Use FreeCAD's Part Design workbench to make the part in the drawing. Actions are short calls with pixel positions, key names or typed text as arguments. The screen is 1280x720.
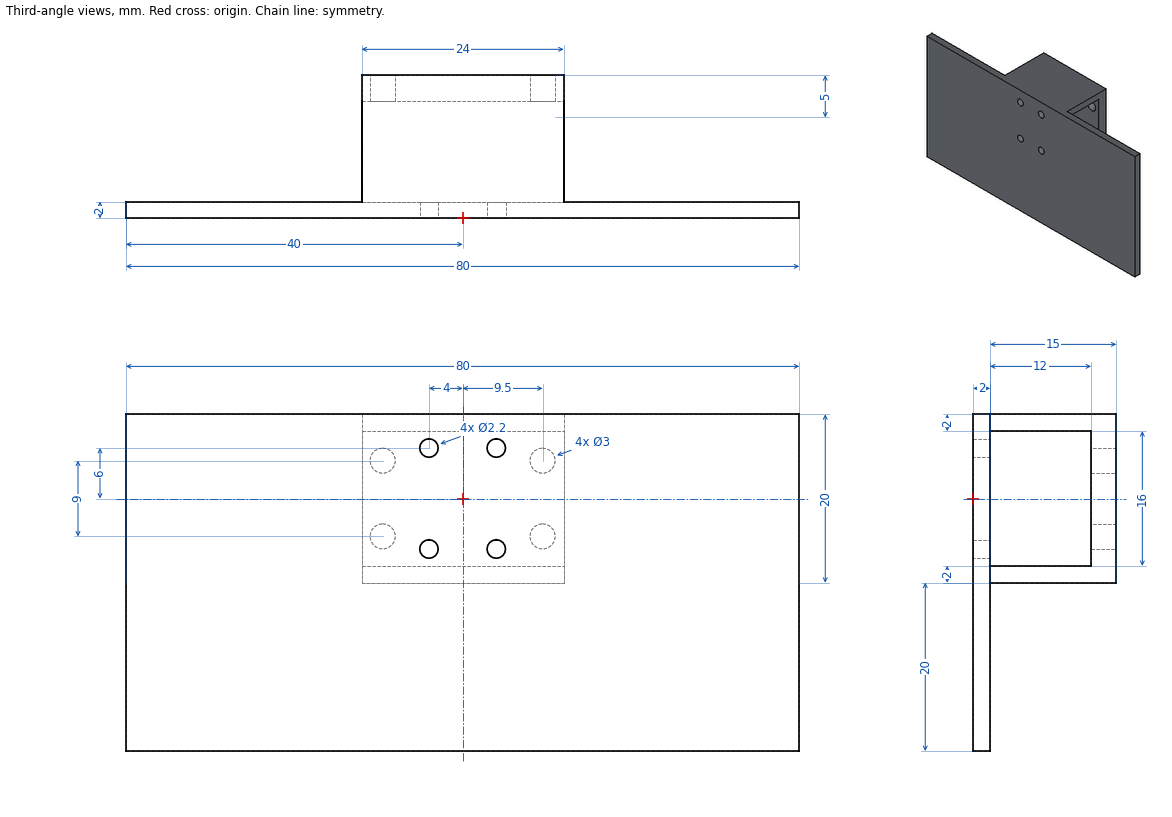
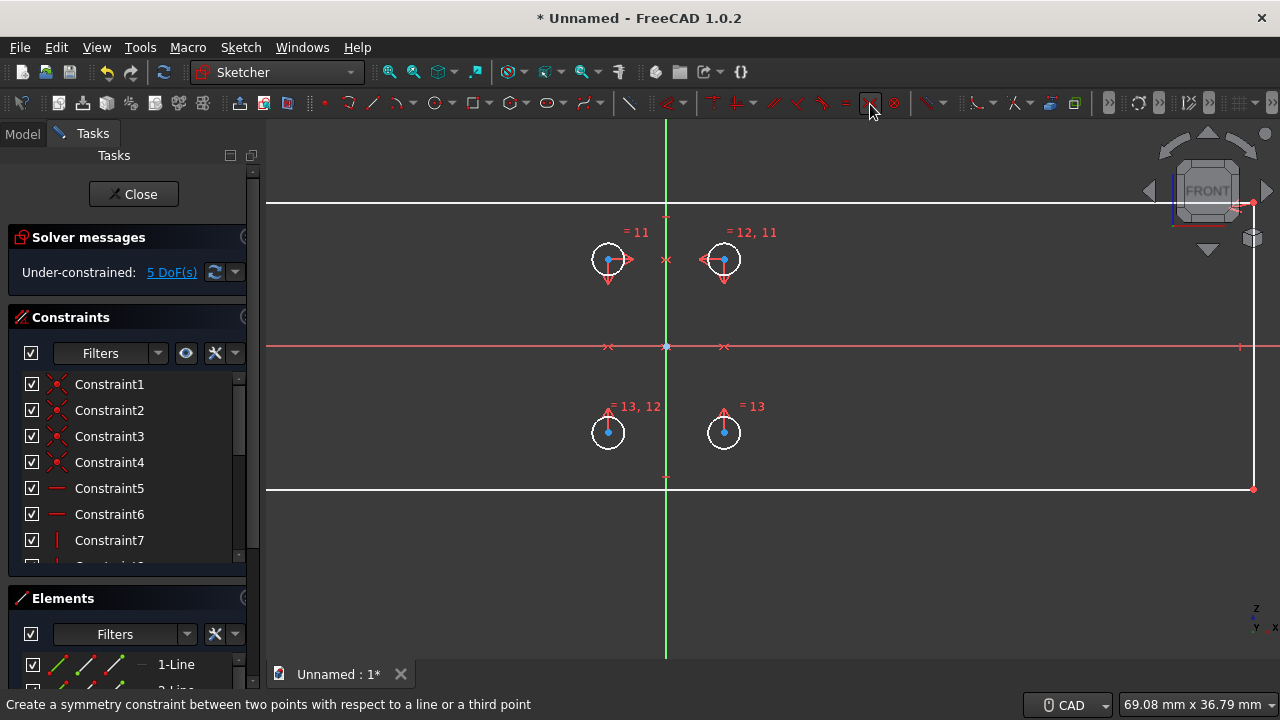
scroll(620, 248, up, 2)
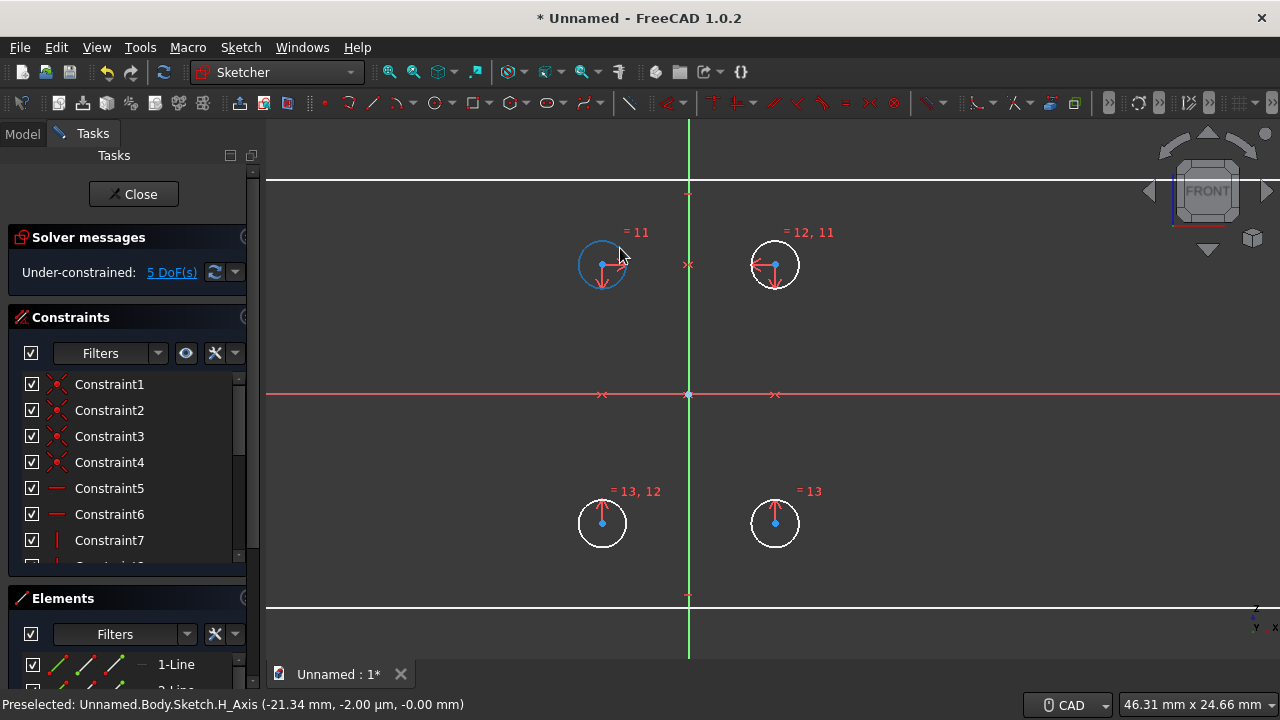
click(619, 248)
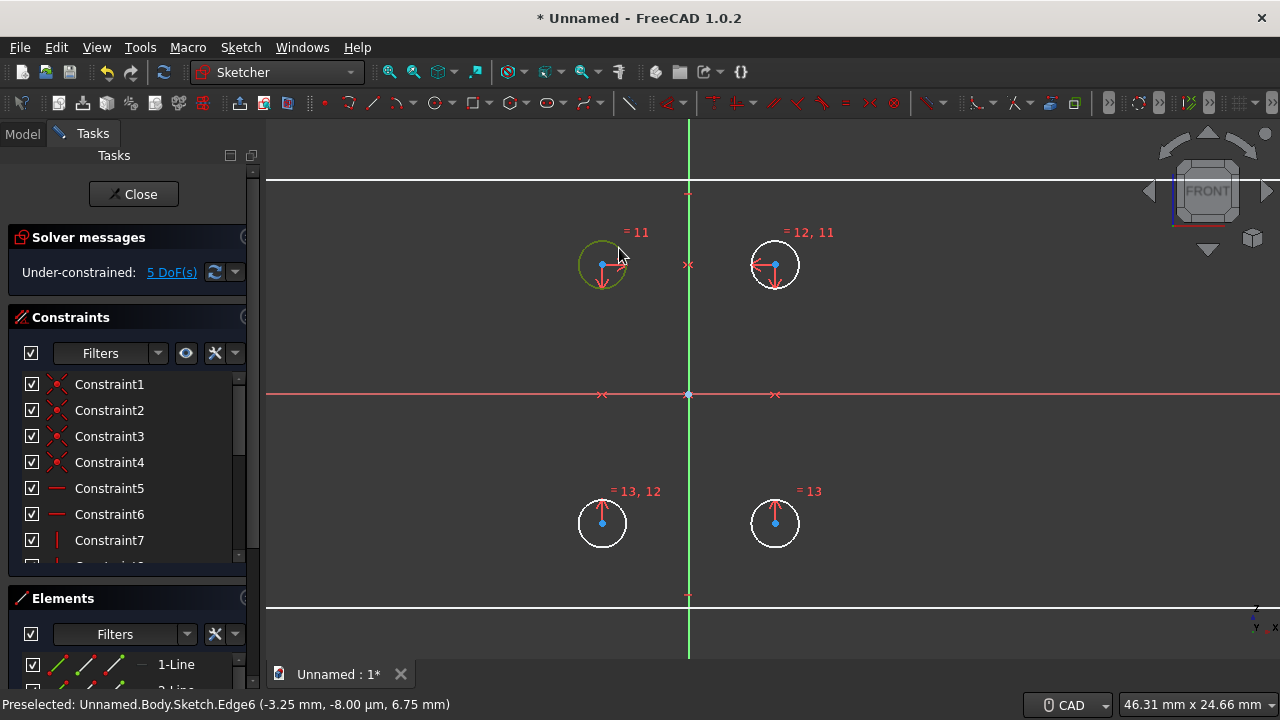
key(k)
key(o)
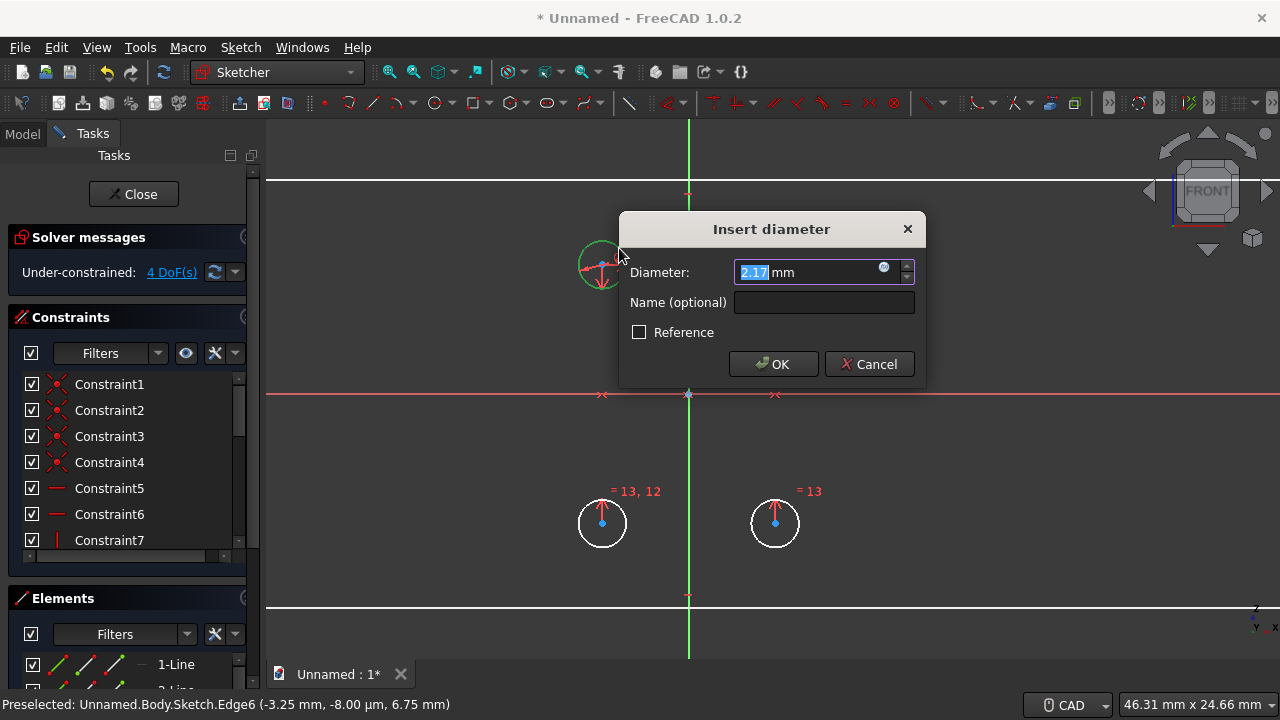
text(2.2)
key(Return)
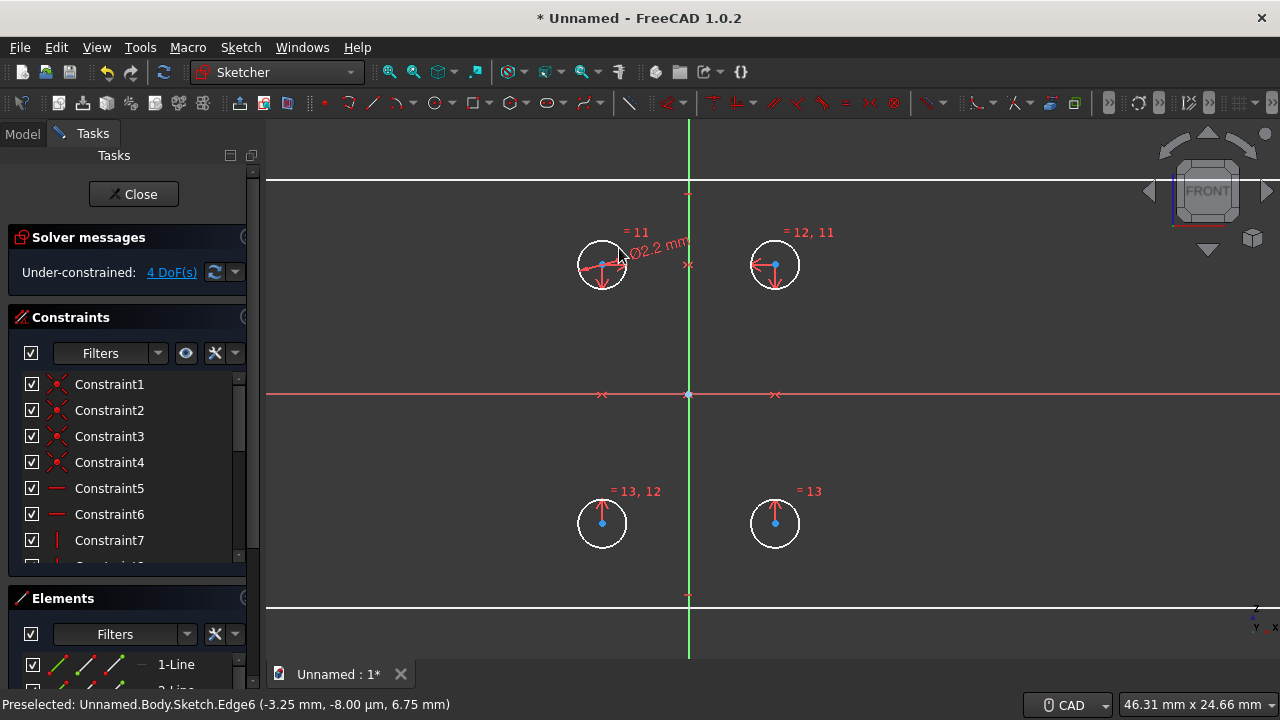
click(602, 265)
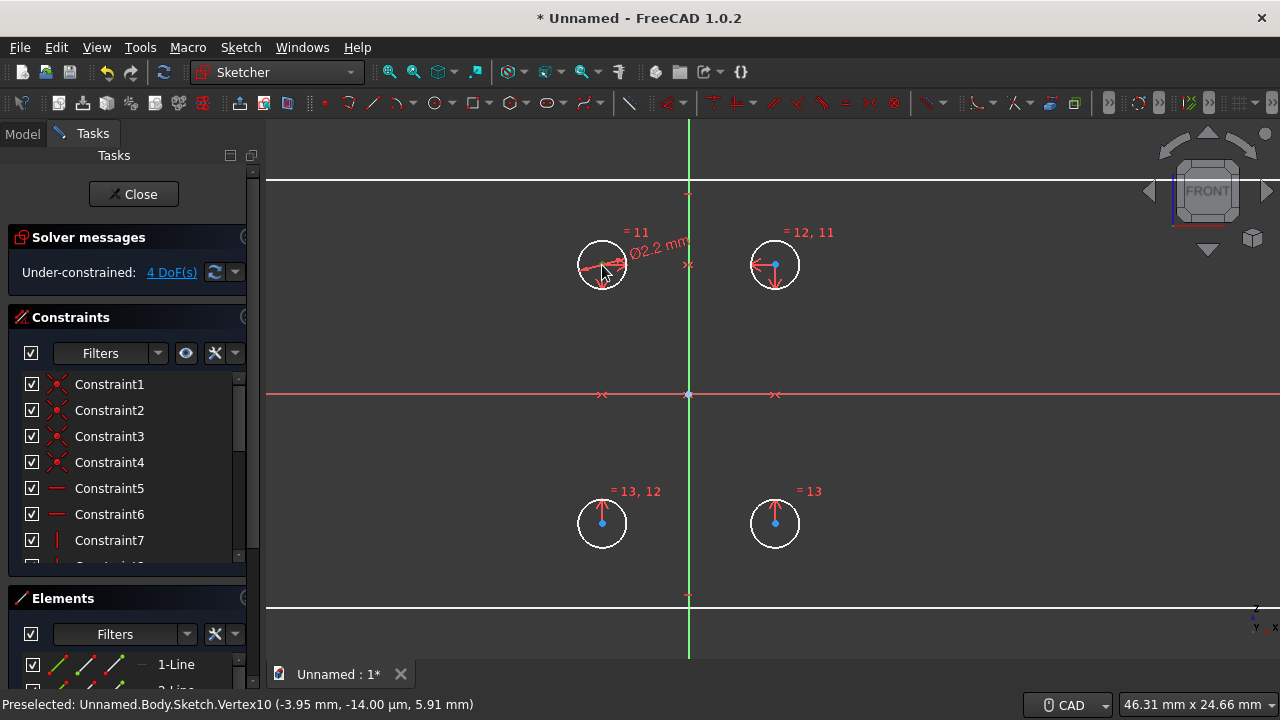
click(686, 104)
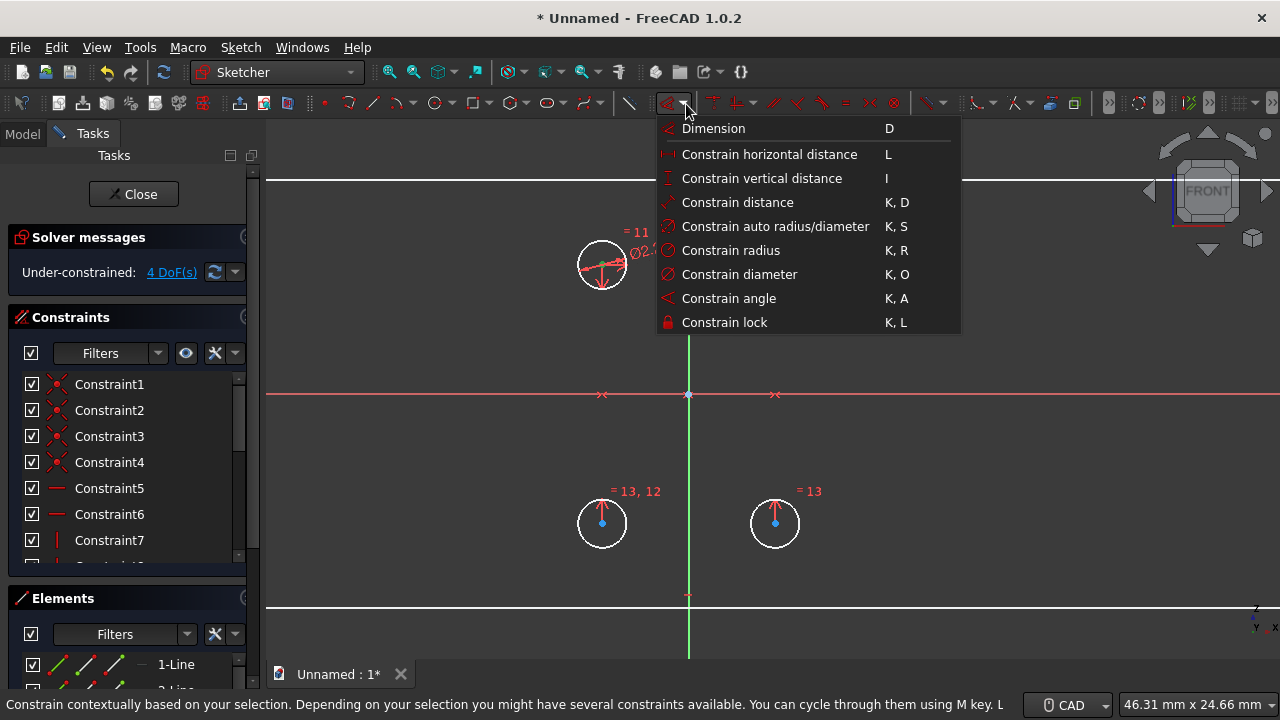
click(809, 154)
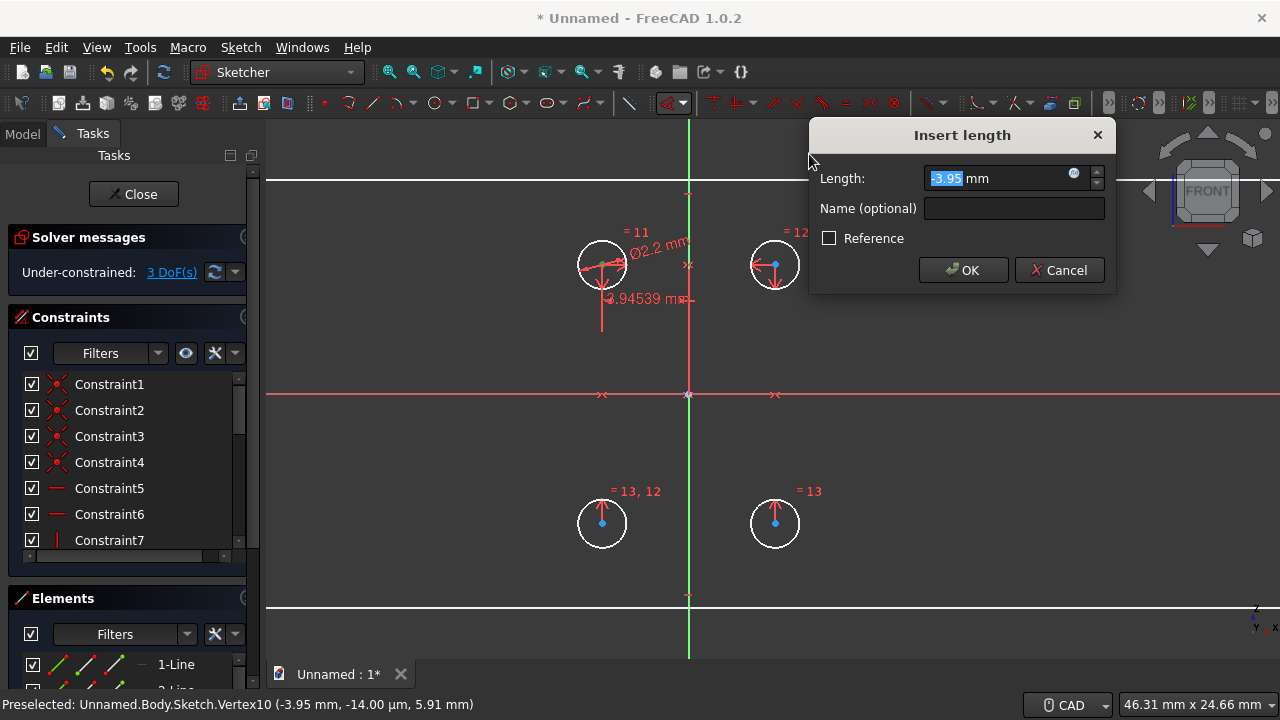
text(-4)
key(Return)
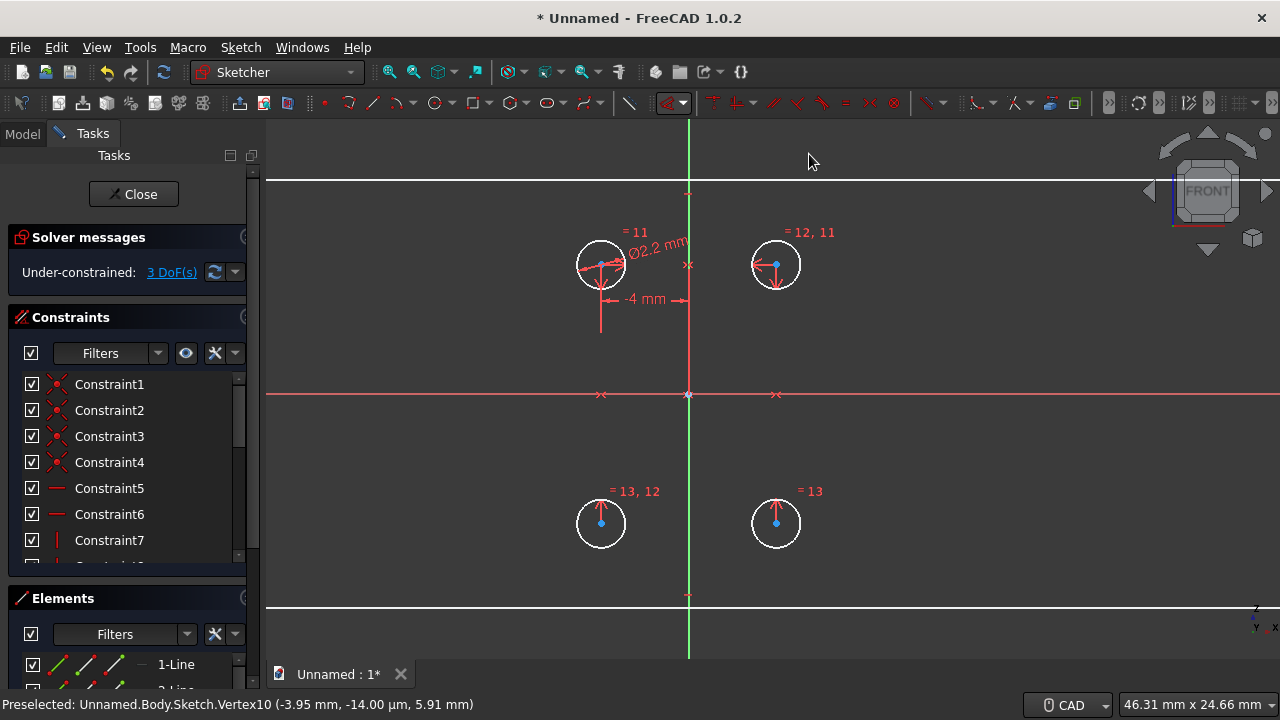
scroll(711, 387, down, 6)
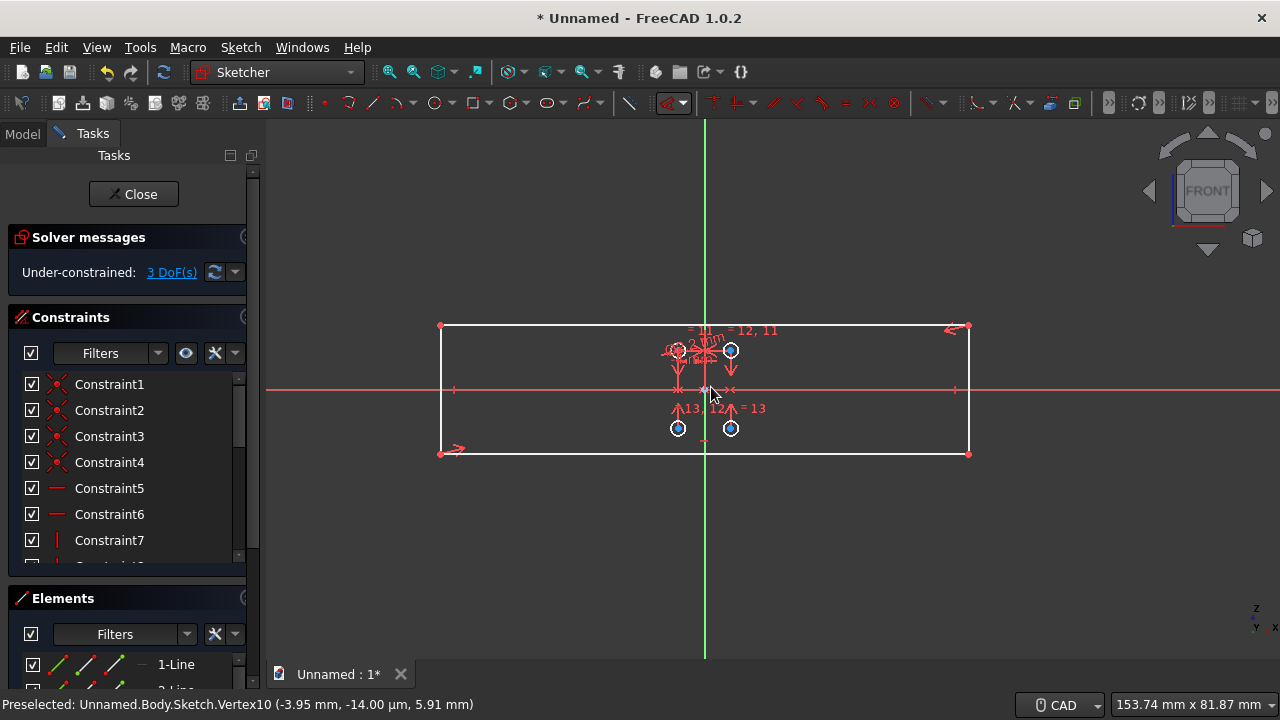
click(678, 351)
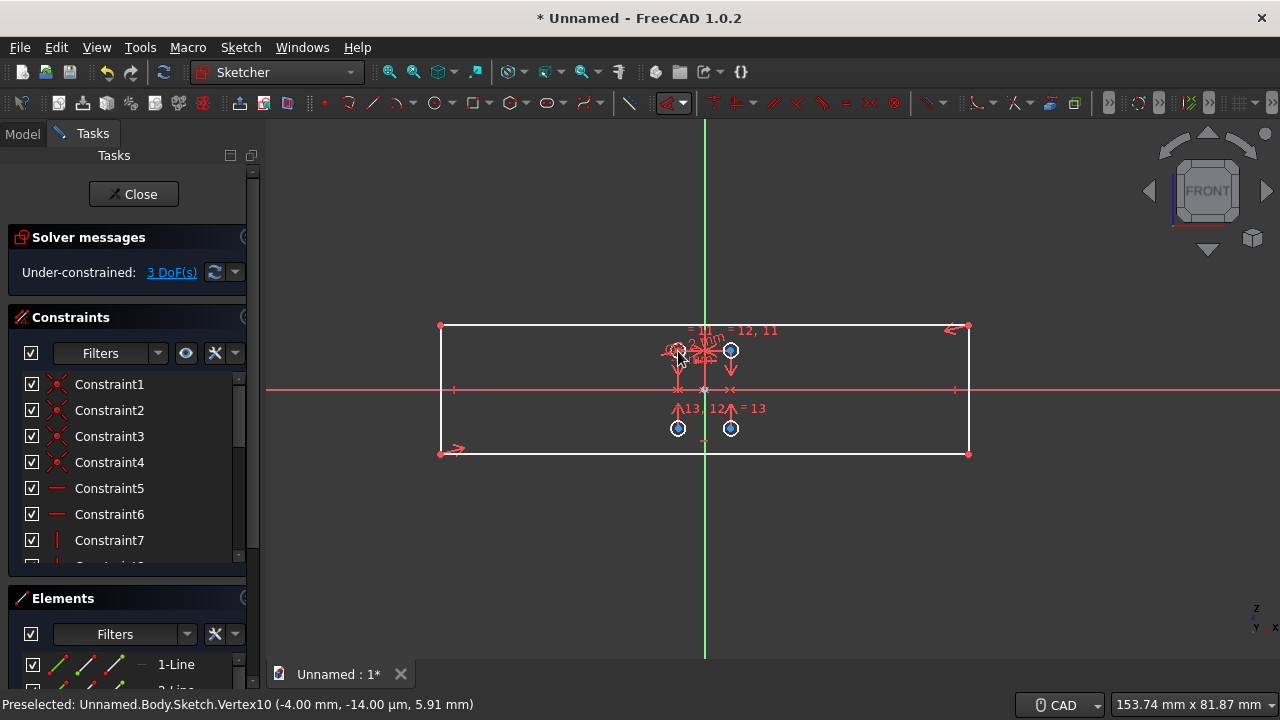
key(i)